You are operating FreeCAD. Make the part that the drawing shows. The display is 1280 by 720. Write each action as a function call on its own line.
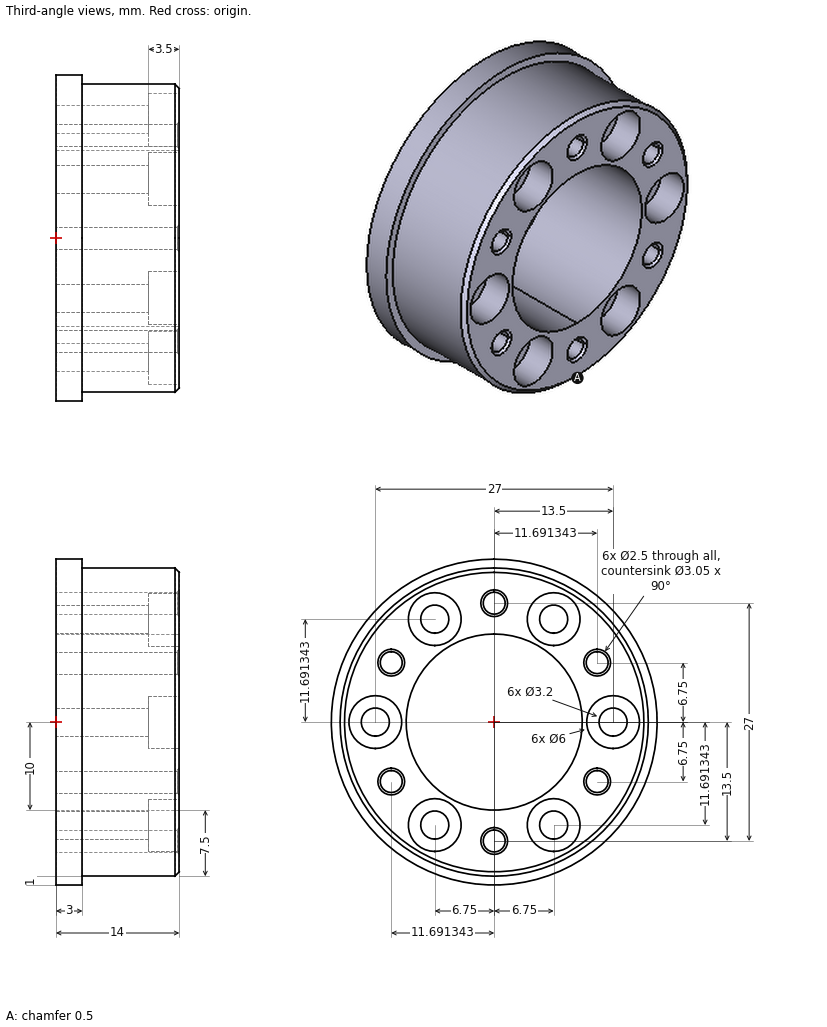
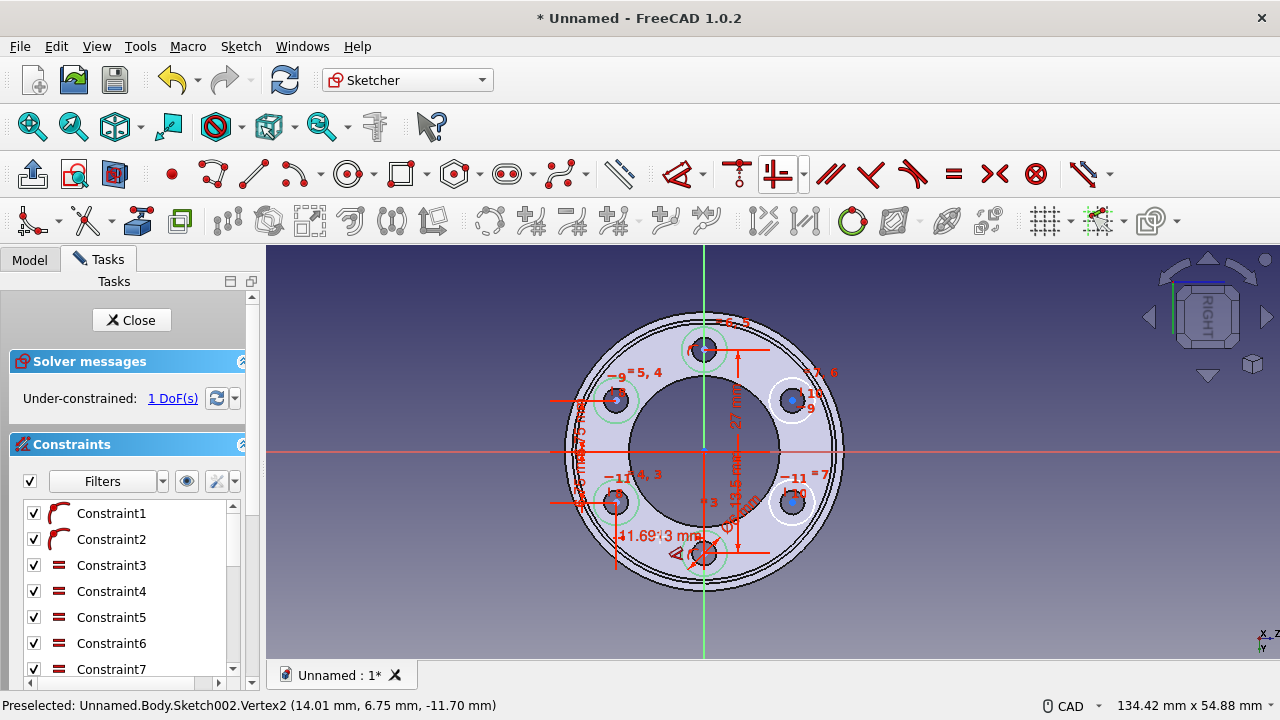
click(792, 401)
click(748, 367)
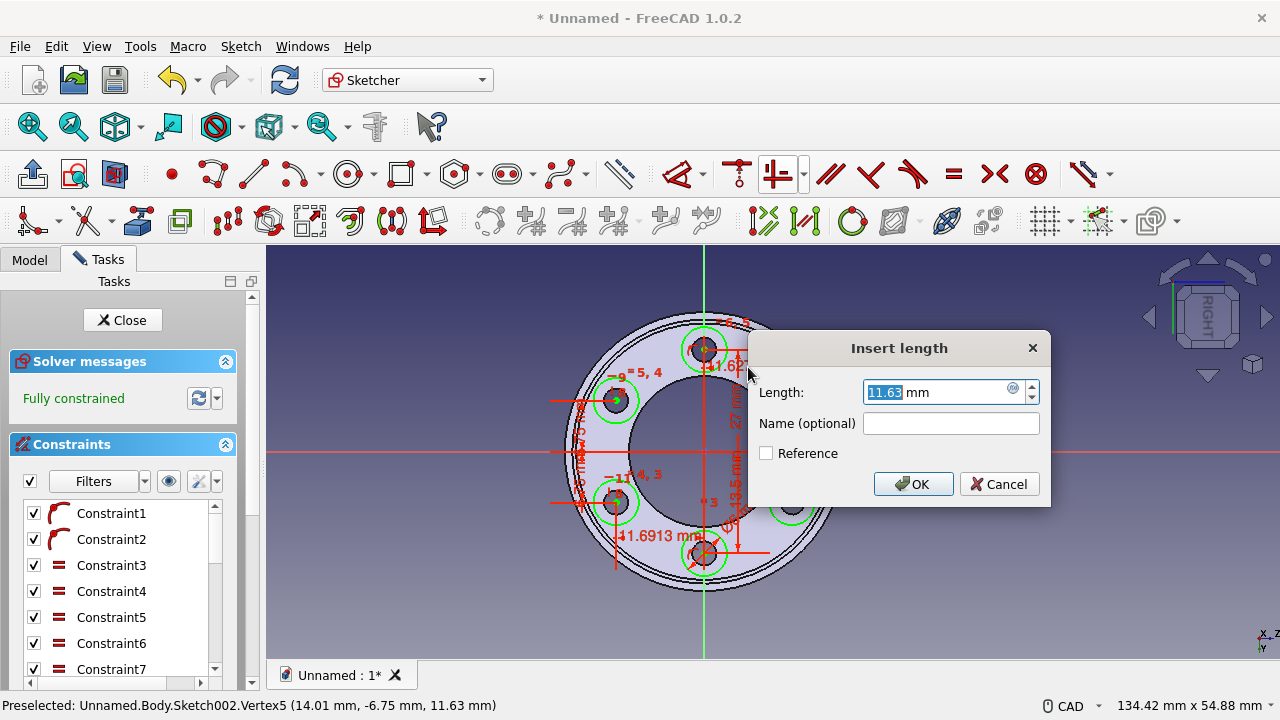
text(11.691343)
key(Return)
key(Escape)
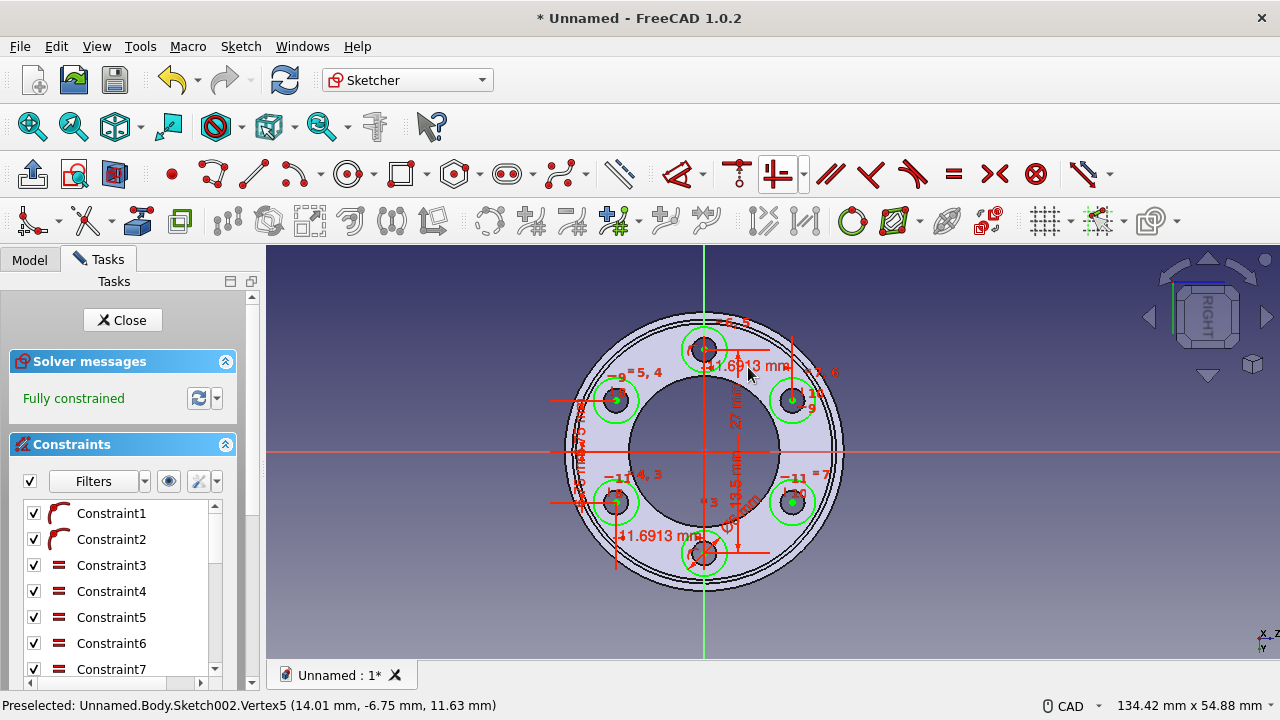
click(123, 320)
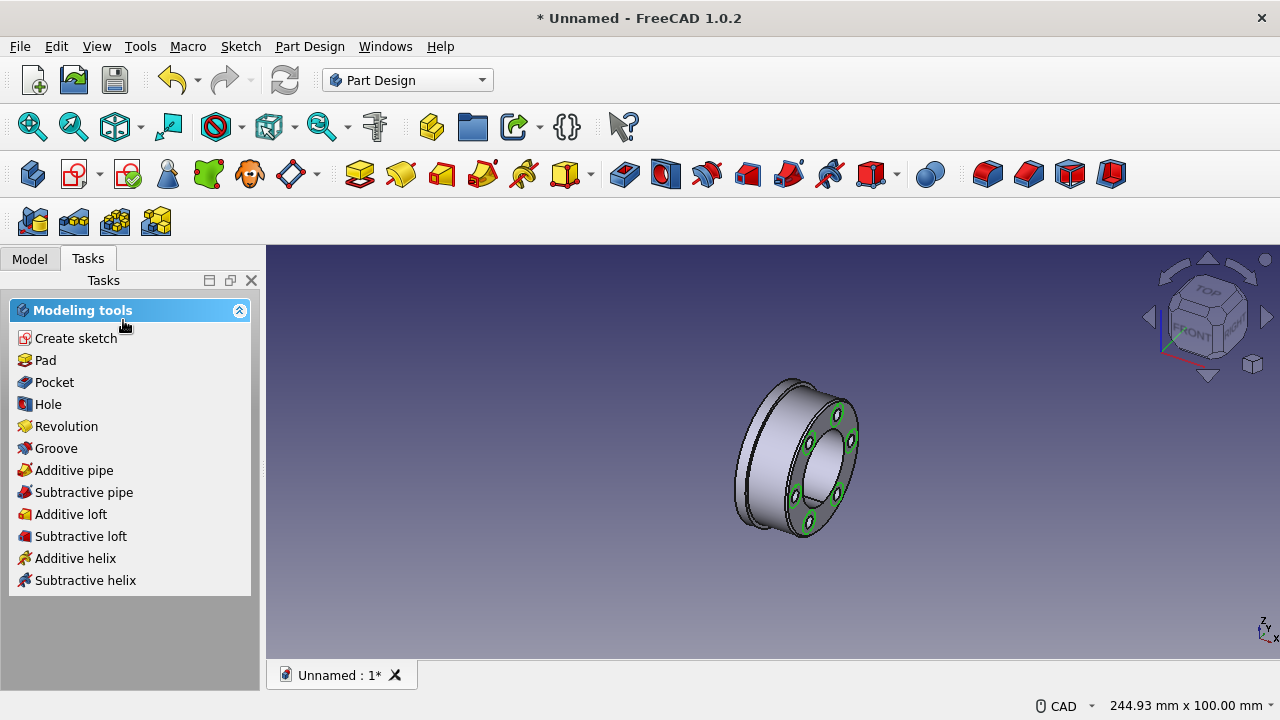
click(625, 174)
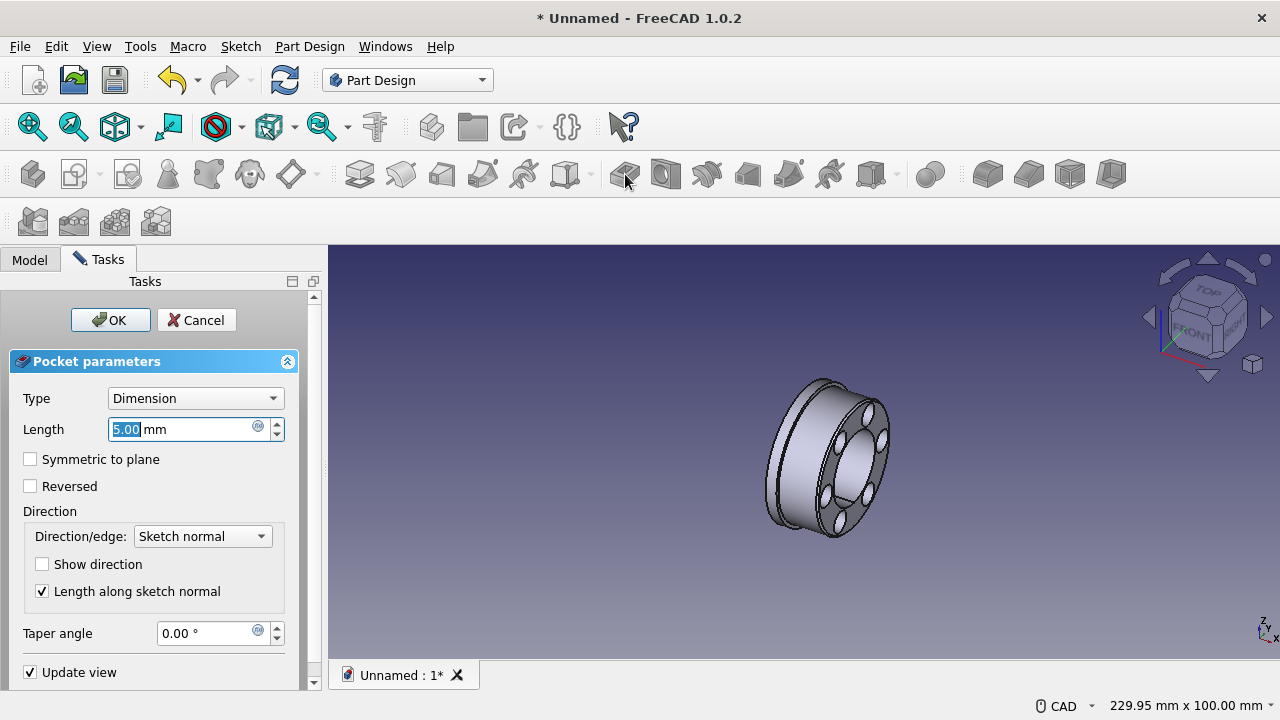
text(3.5)
key(Tab)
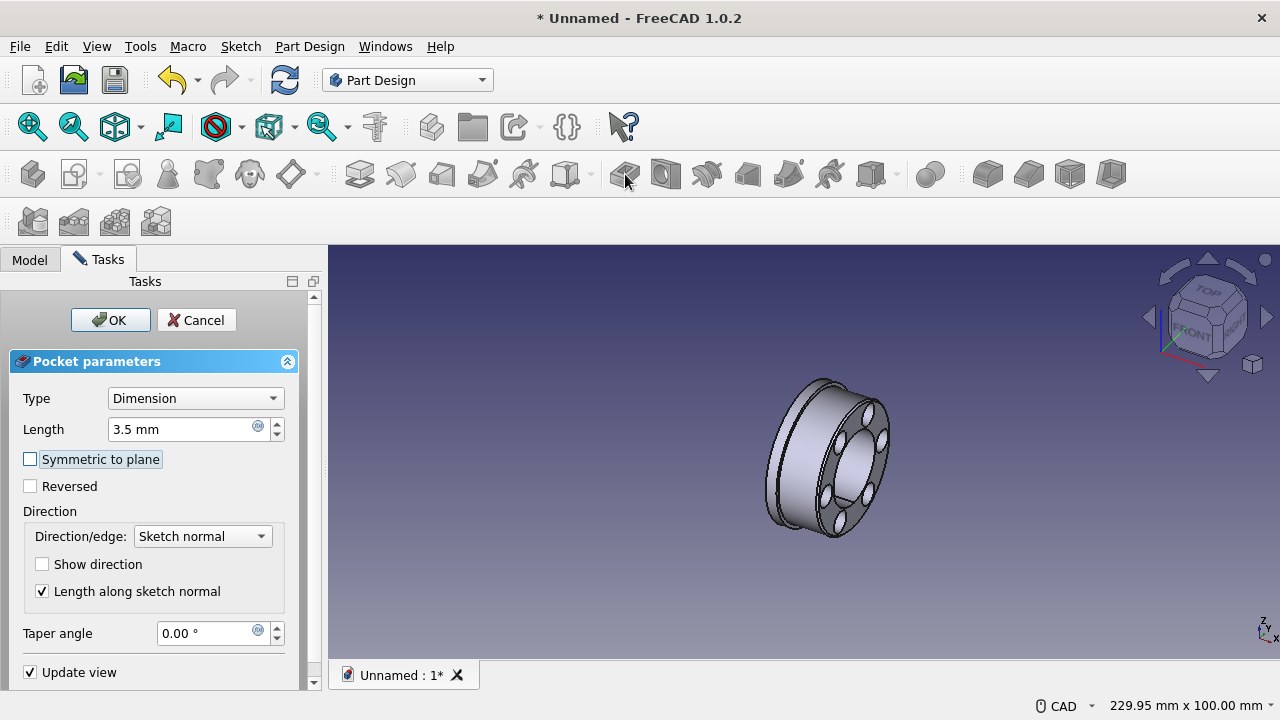
click(111, 320)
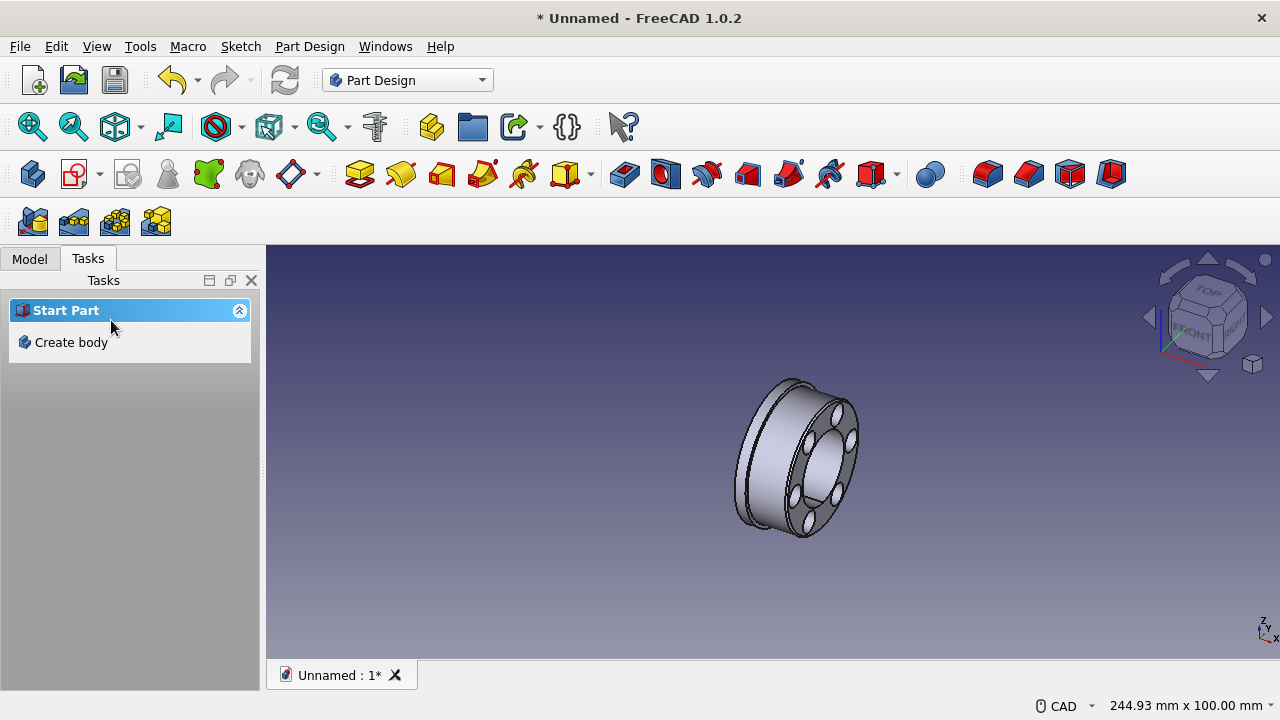
click(853, 421)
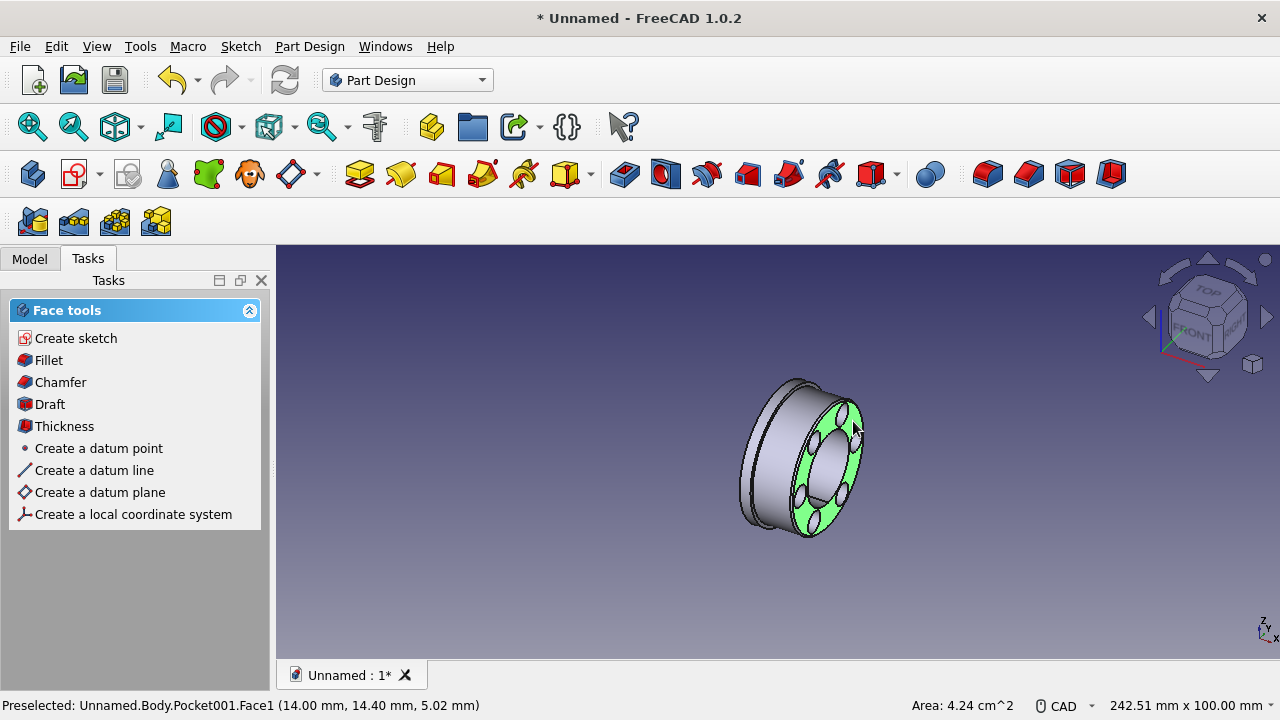
click(74, 174)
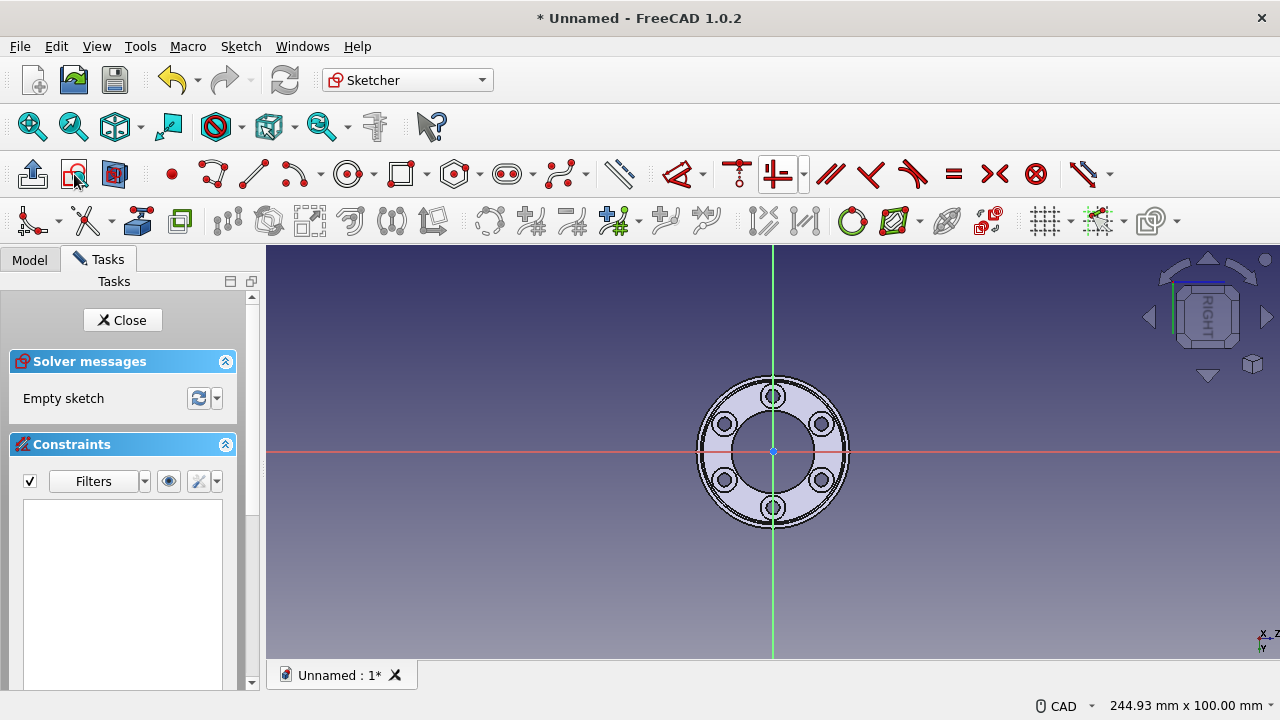
scroll(829, 452, up, 4)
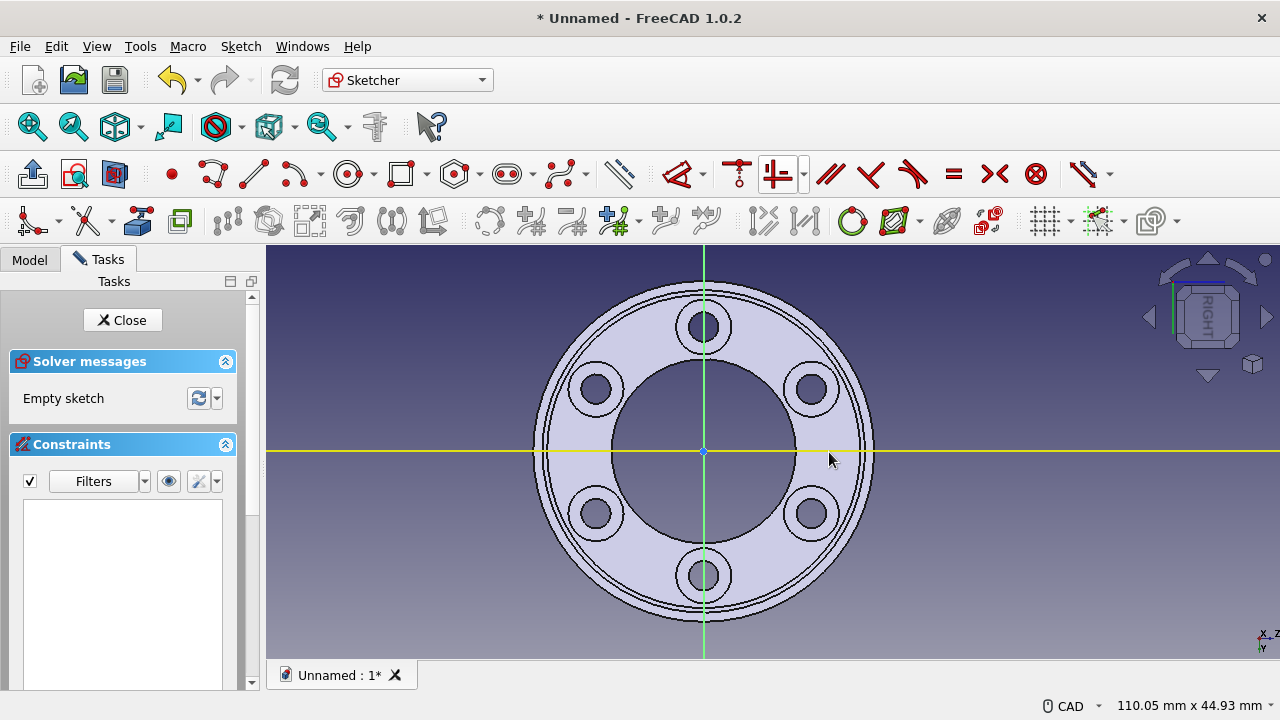
click(348, 174)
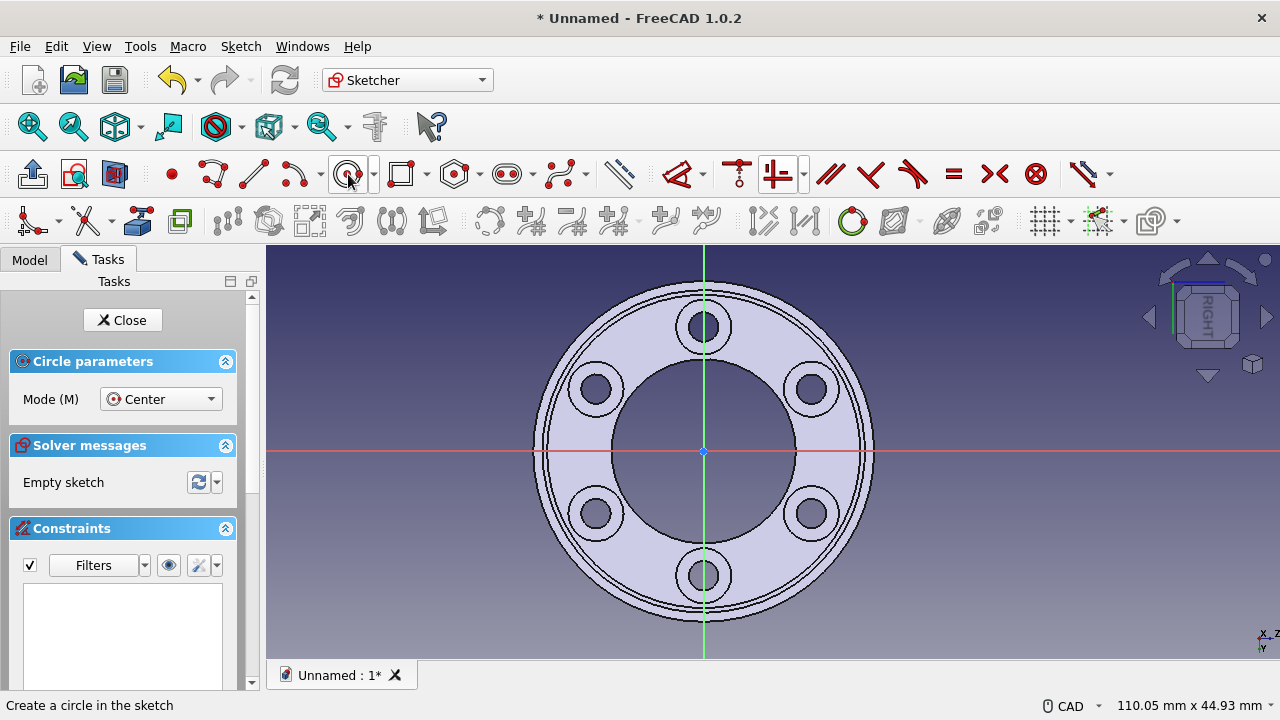
scroll(766, 559, up, 4)